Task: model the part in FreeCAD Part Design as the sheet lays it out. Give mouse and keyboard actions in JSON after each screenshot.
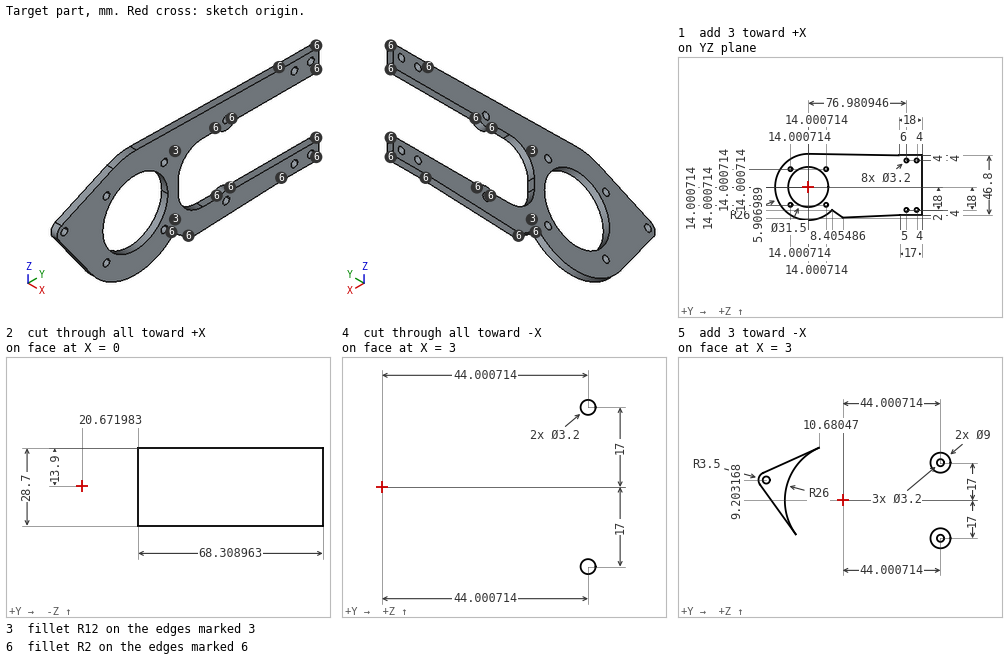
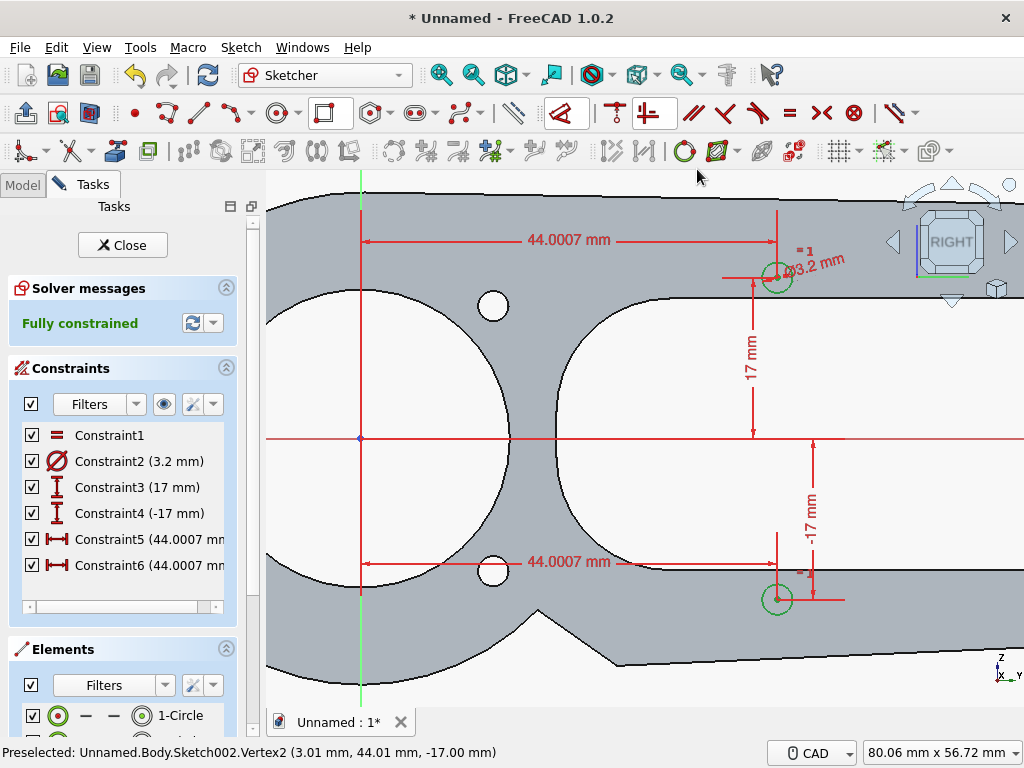
{"action": "left_click", "coordinate": [123, 245]}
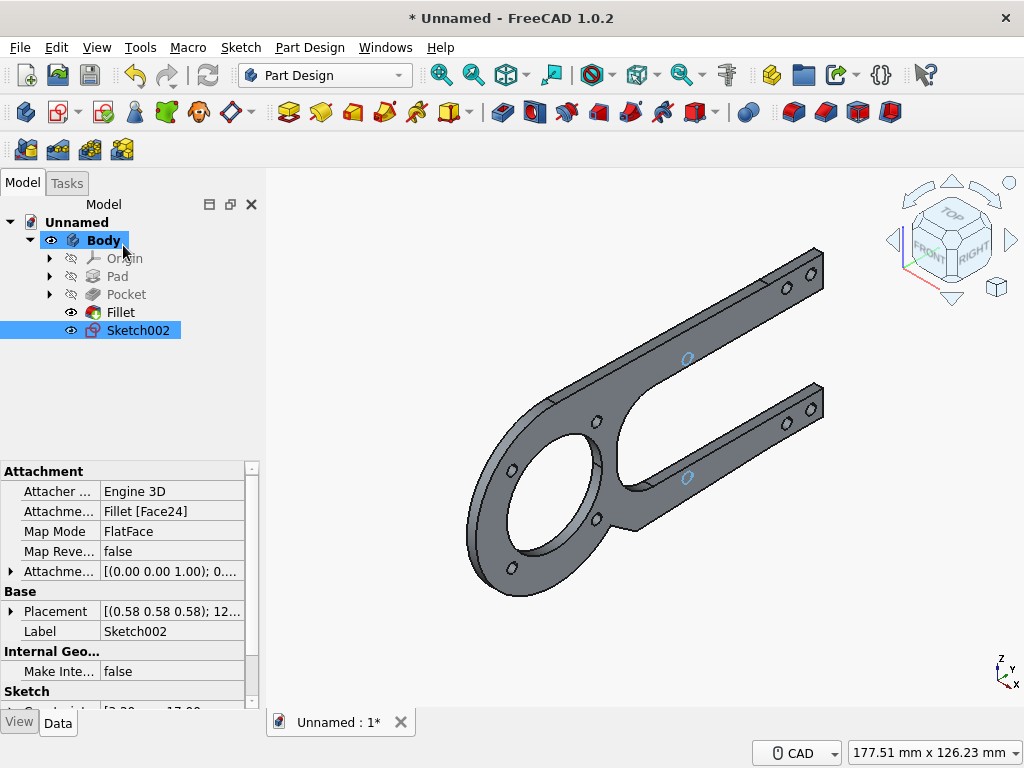
{"action": "left_click", "coordinate": [504, 112]}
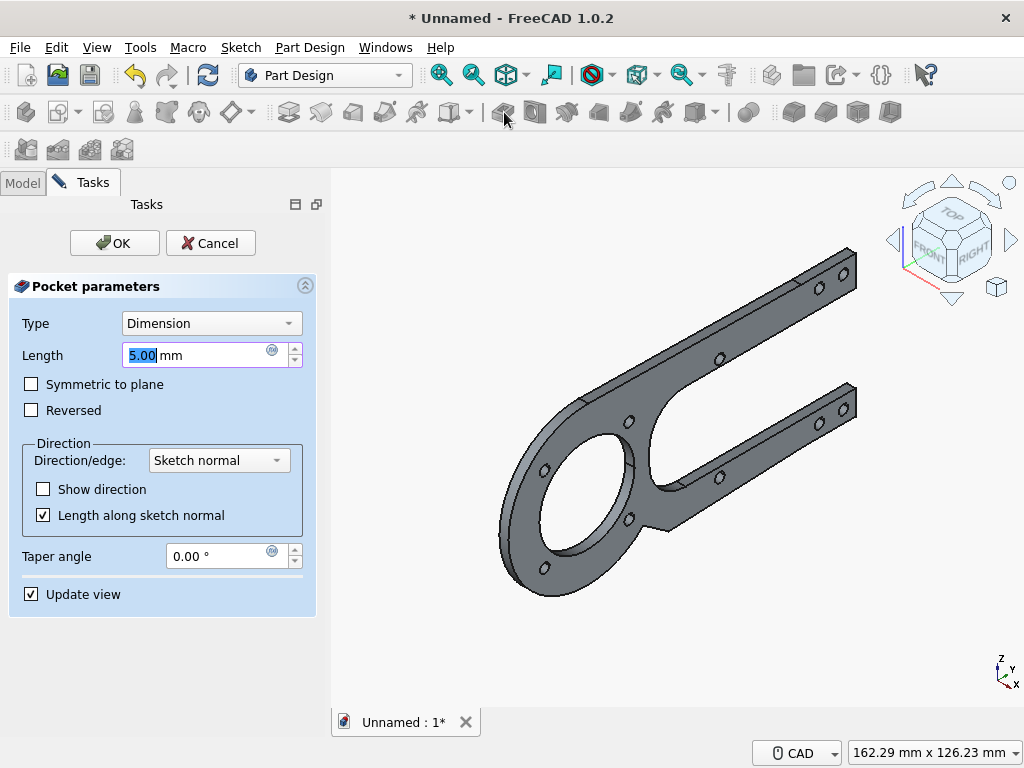
{"action": "left_click", "coordinate": [212, 324]}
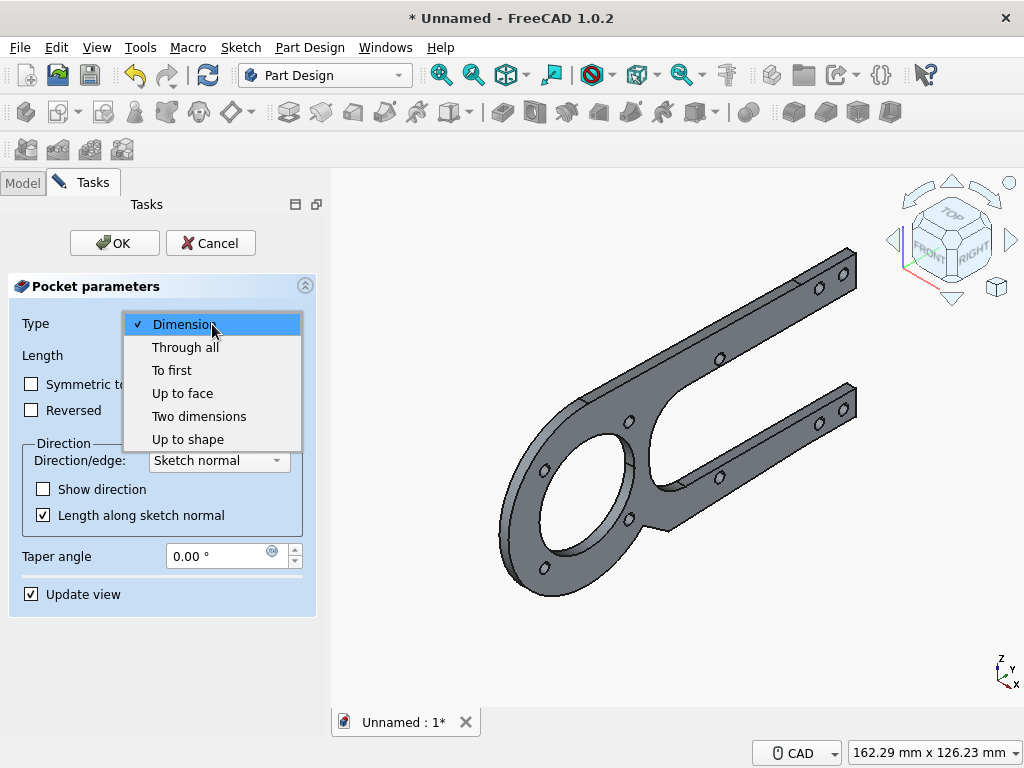
{"action": "left_click", "coordinate": [212, 348]}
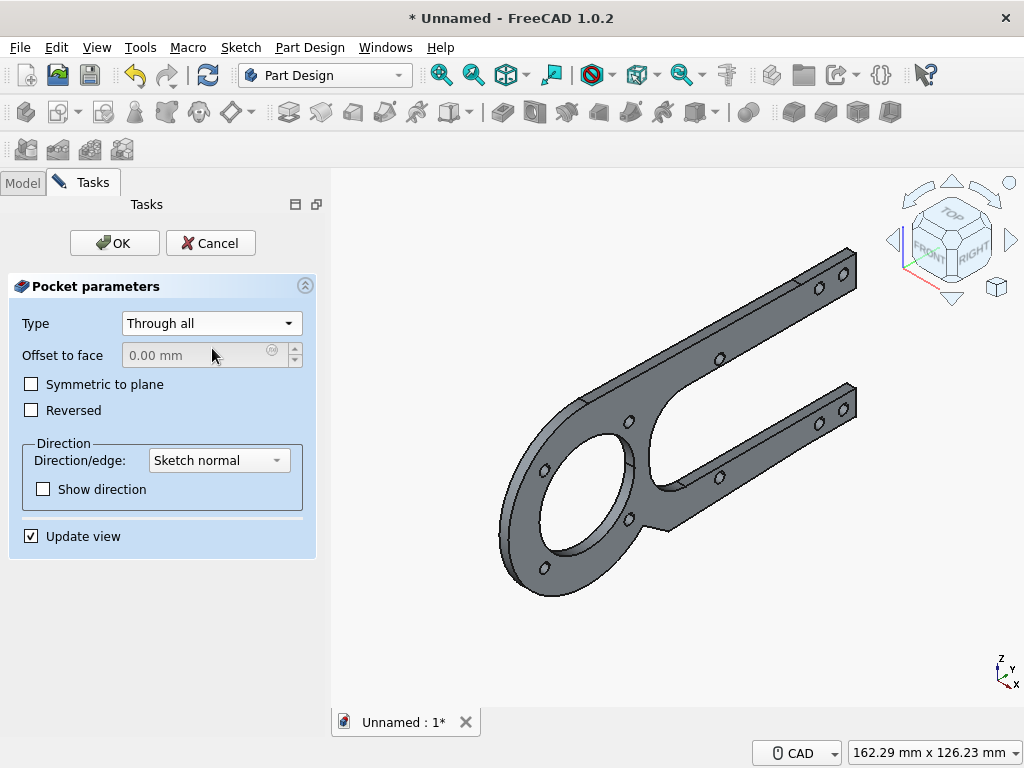
{"action": "left_click", "coordinate": [115, 243]}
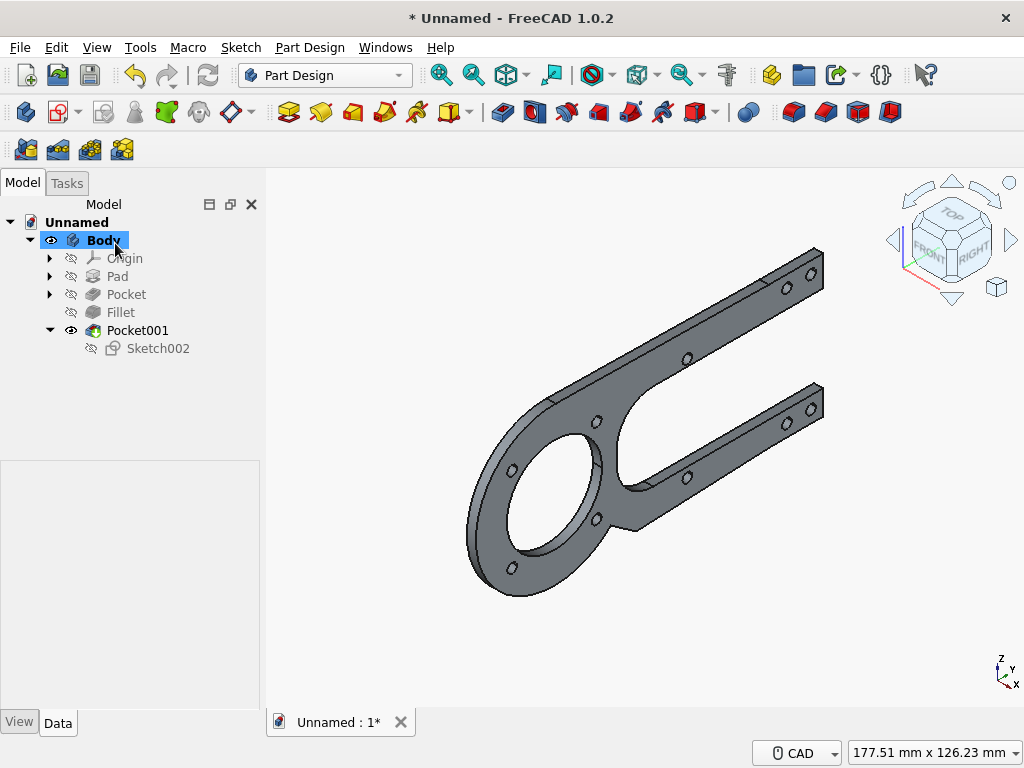
{"action": "left_click", "coordinate": [550, 419]}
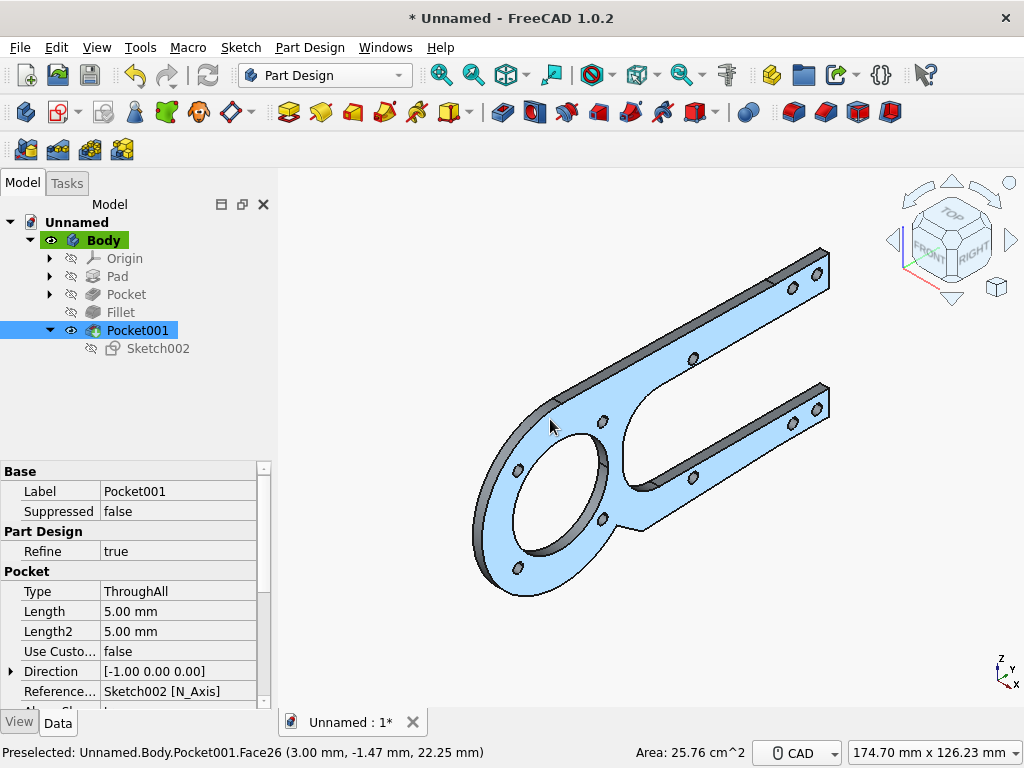
{"action": "left_click", "coordinate": [58, 112]}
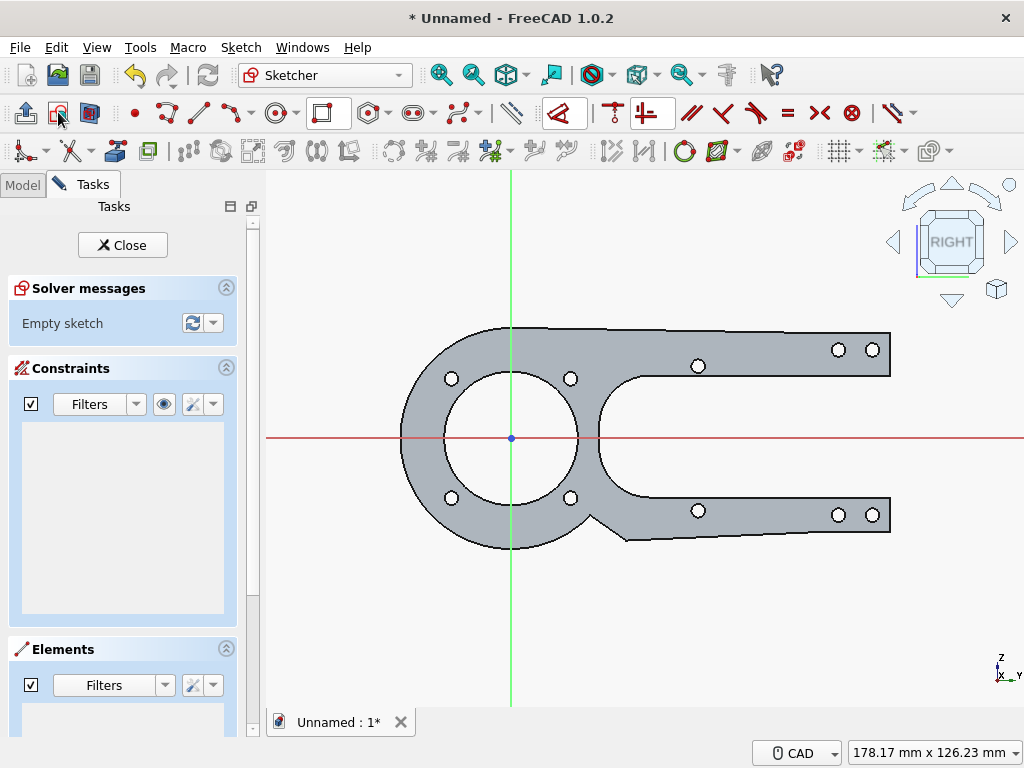
{"action": "left_click", "coordinate": [200, 114]}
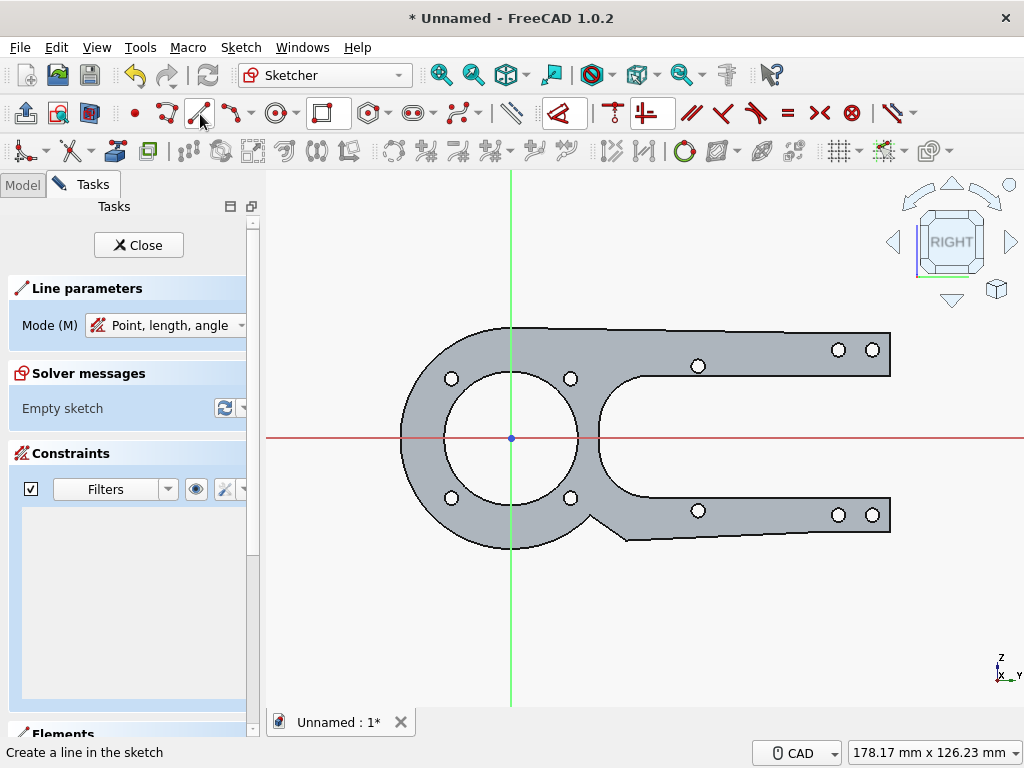
{"action": "left_click", "coordinate": [466, 338]}
{"action": "left_click", "coordinate": [359, 386]}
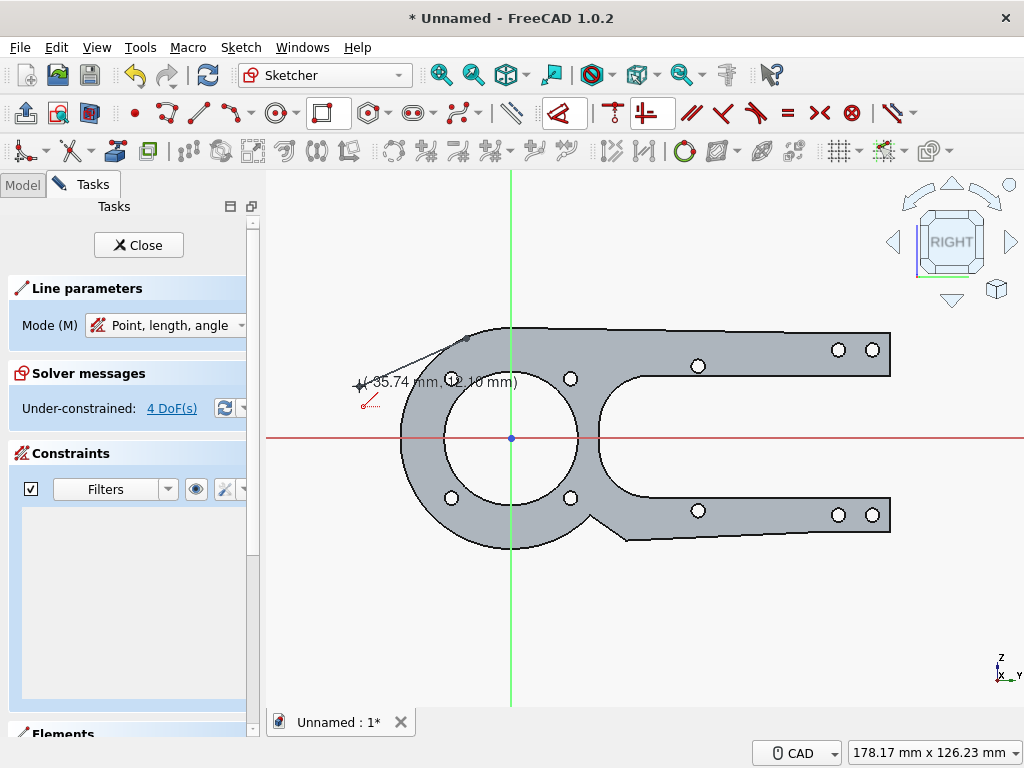
{"action": "left_click", "coordinate": [353, 408]}
{"action": "left_click", "coordinate": [421, 503]}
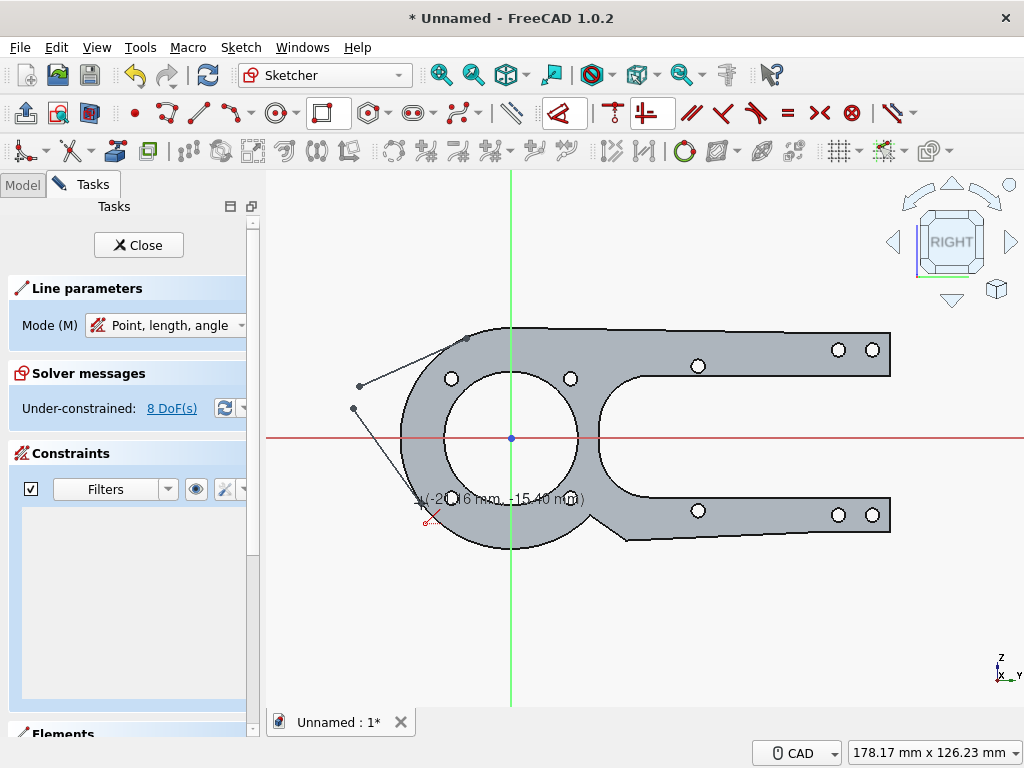
{"action": "left_click", "coordinate": [232, 114]}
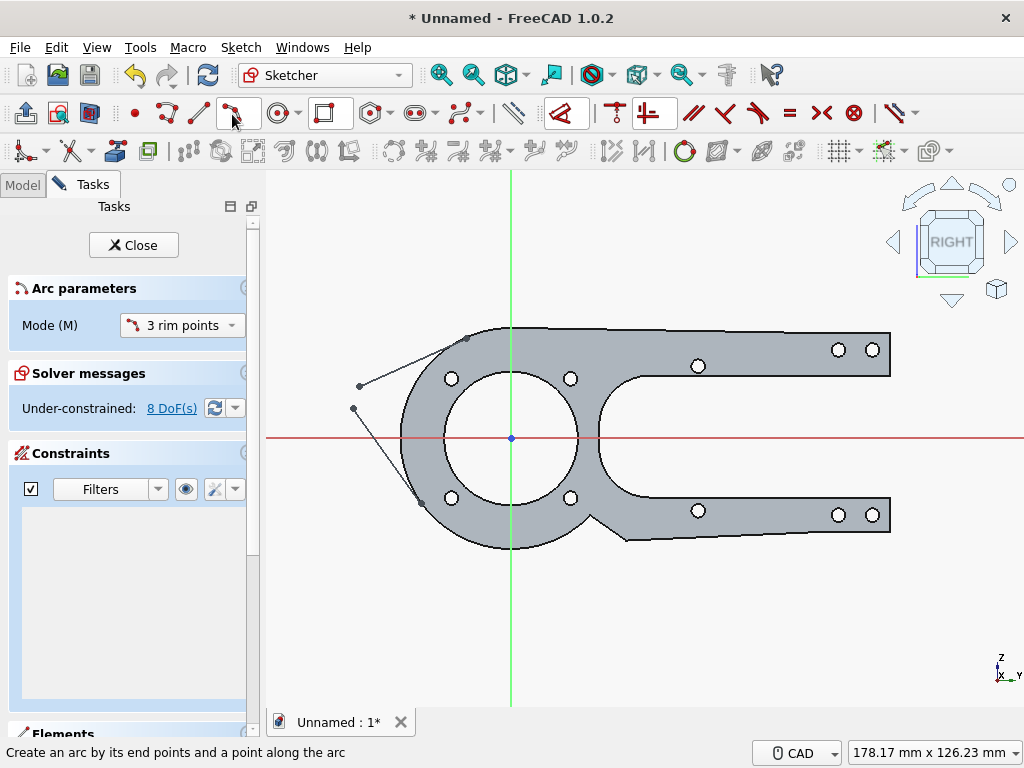
{"action": "left_click", "coordinate": [359, 387]}
{"action": "left_click", "coordinate": [353, 409]}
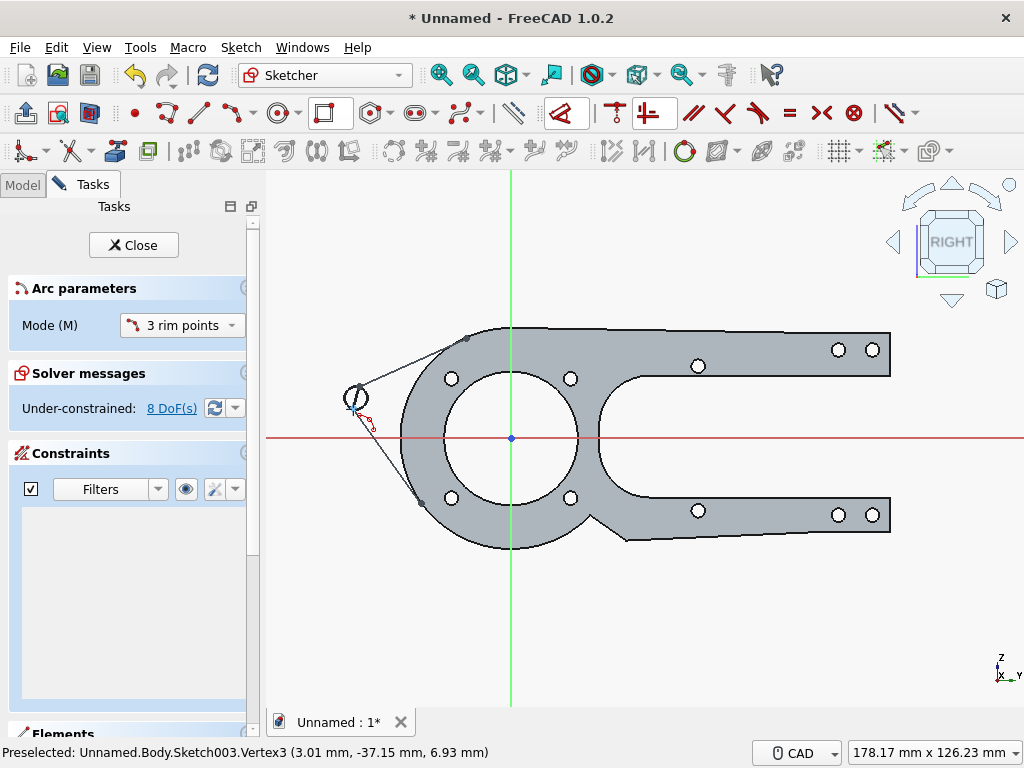
{"action": "scroll", "coordinate": [351, 395], "scroll_direction": "up", "scroll_amount": 6}